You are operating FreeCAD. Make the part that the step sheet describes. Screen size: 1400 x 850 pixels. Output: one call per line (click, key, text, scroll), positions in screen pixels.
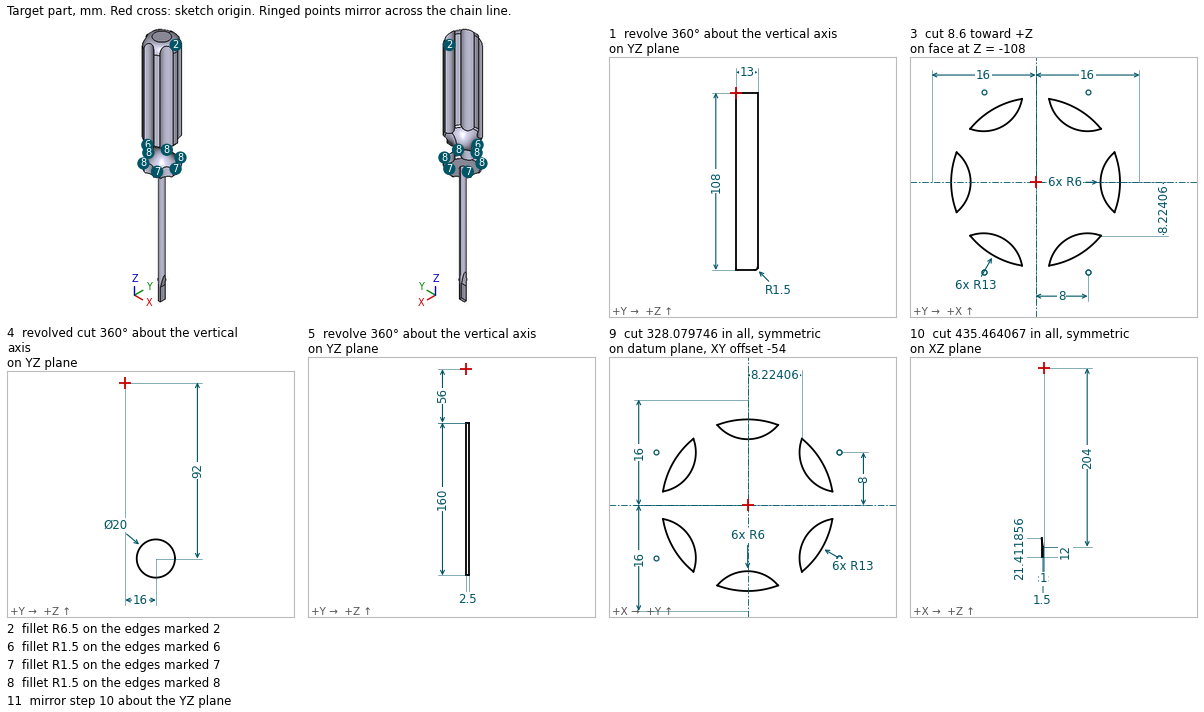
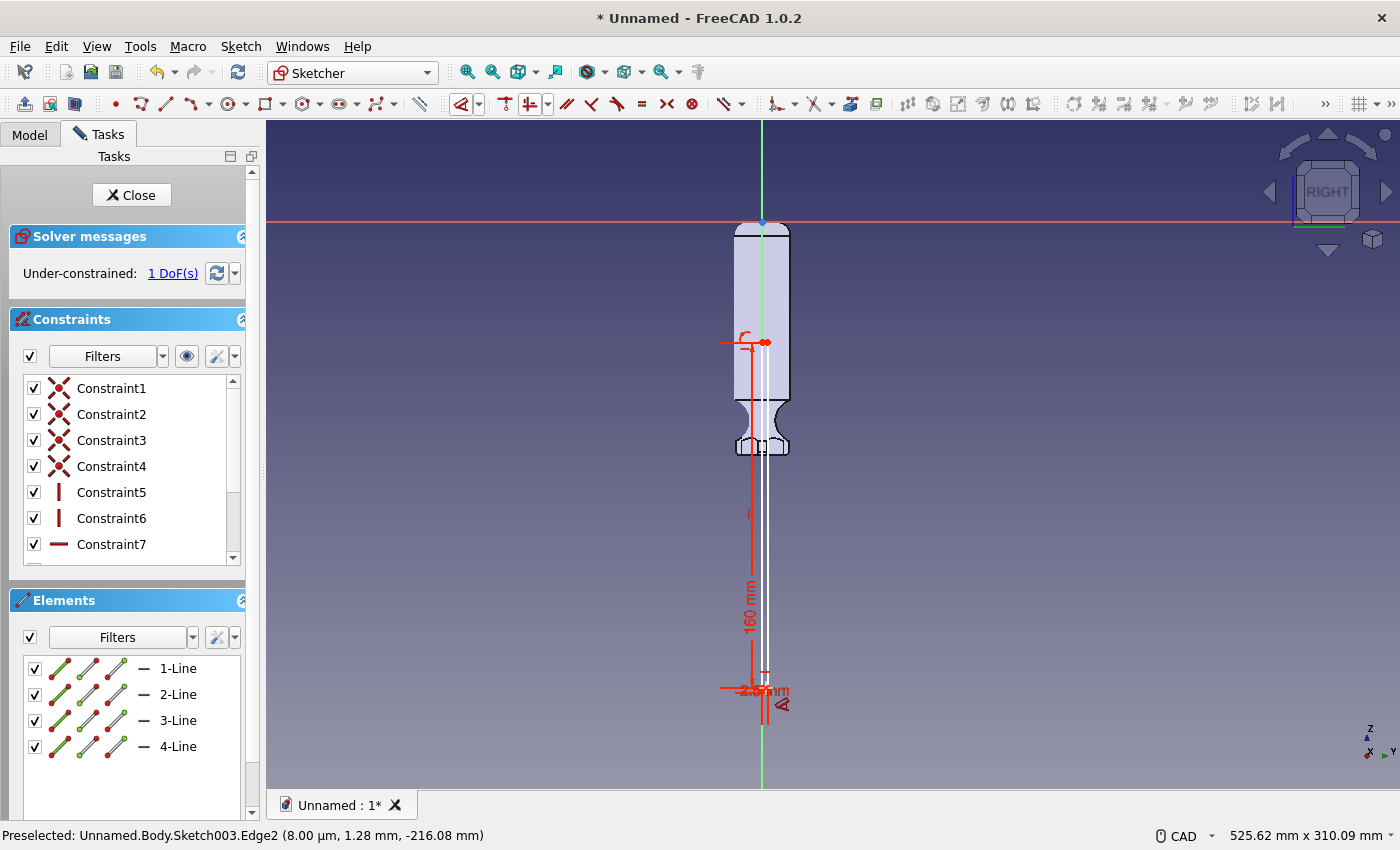
scroll(762, 343, up, 5)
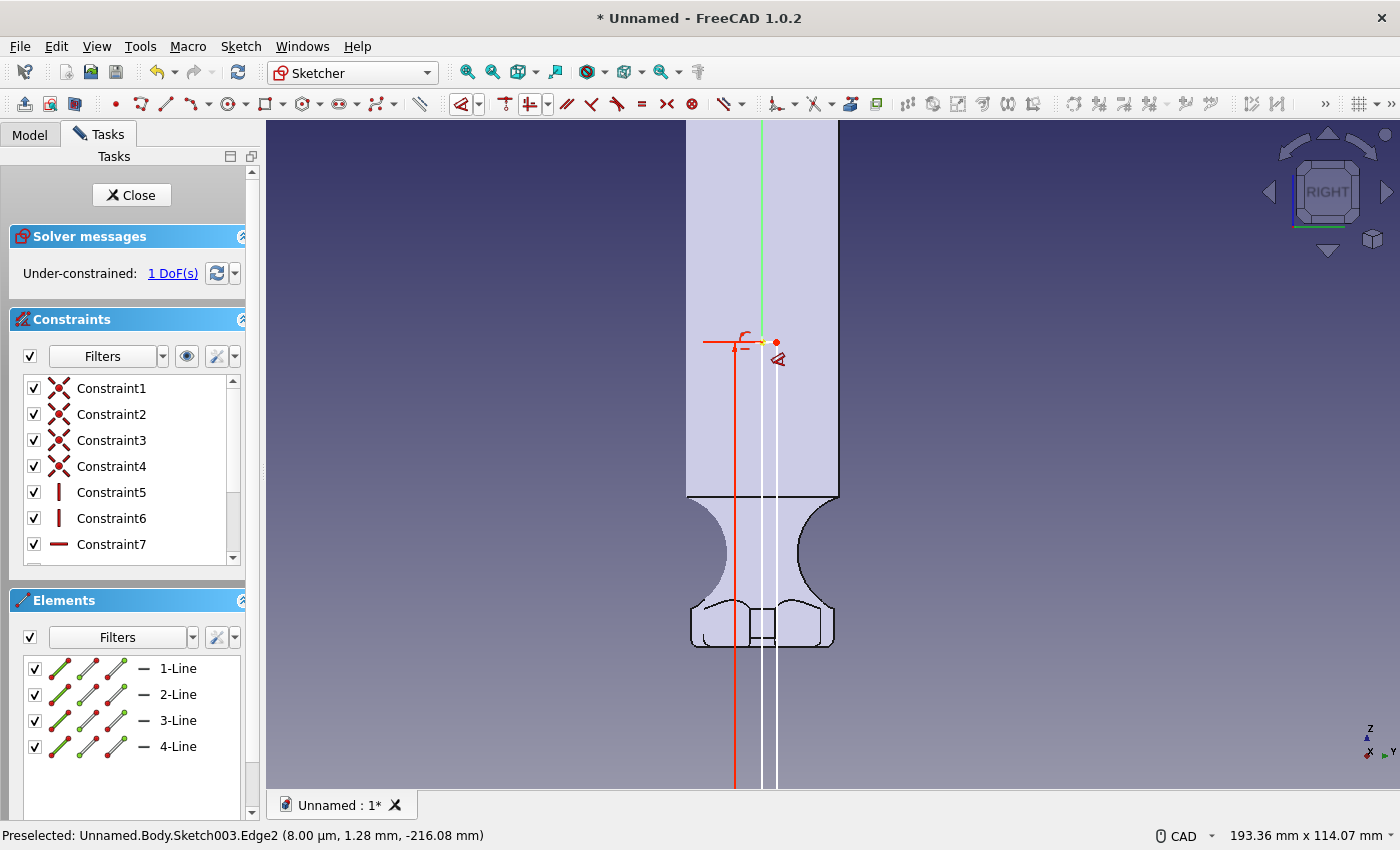
click(762, 342)
click(728, 245)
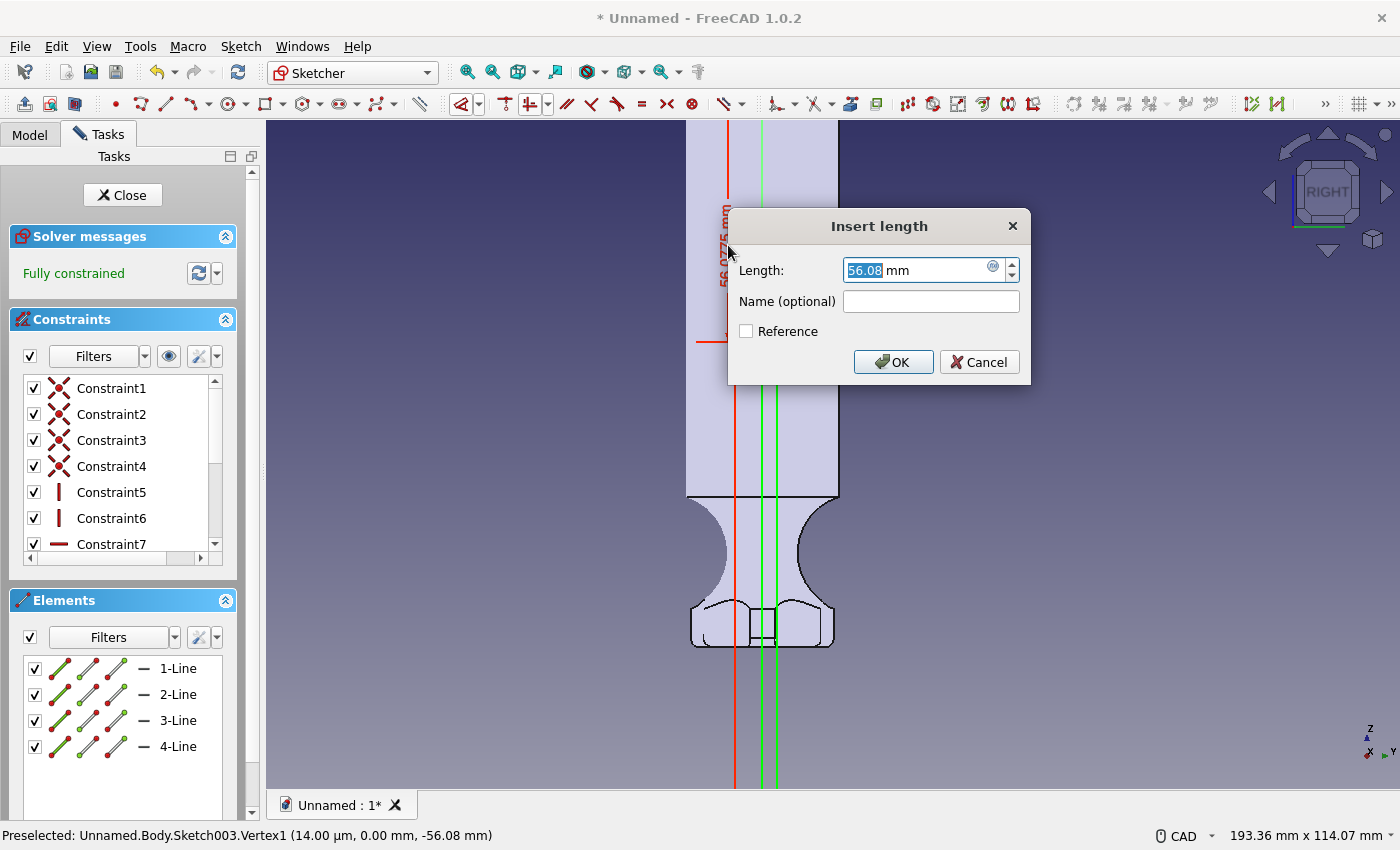
text(56)
key(Return)
key(Escape)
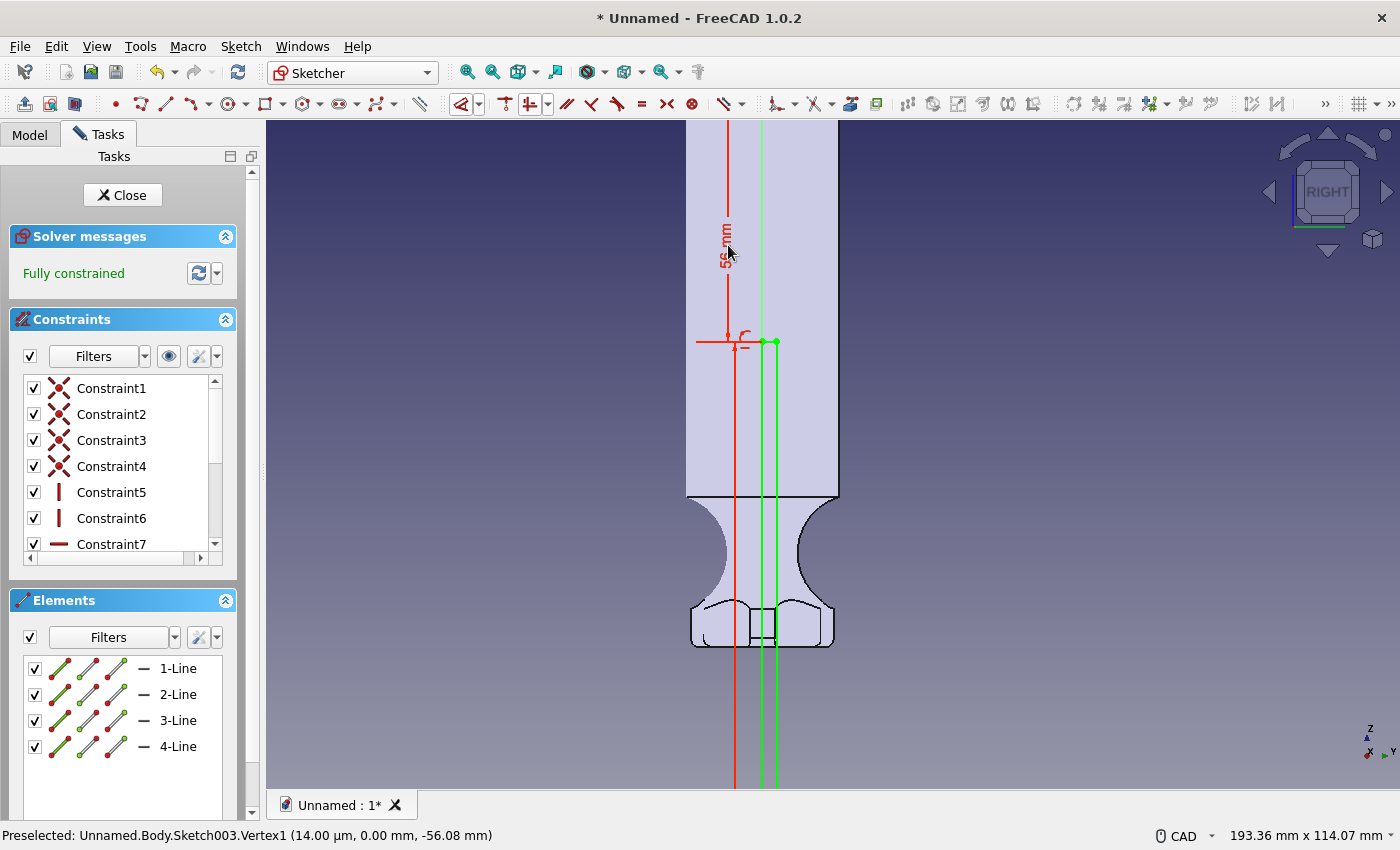
click(123, 195)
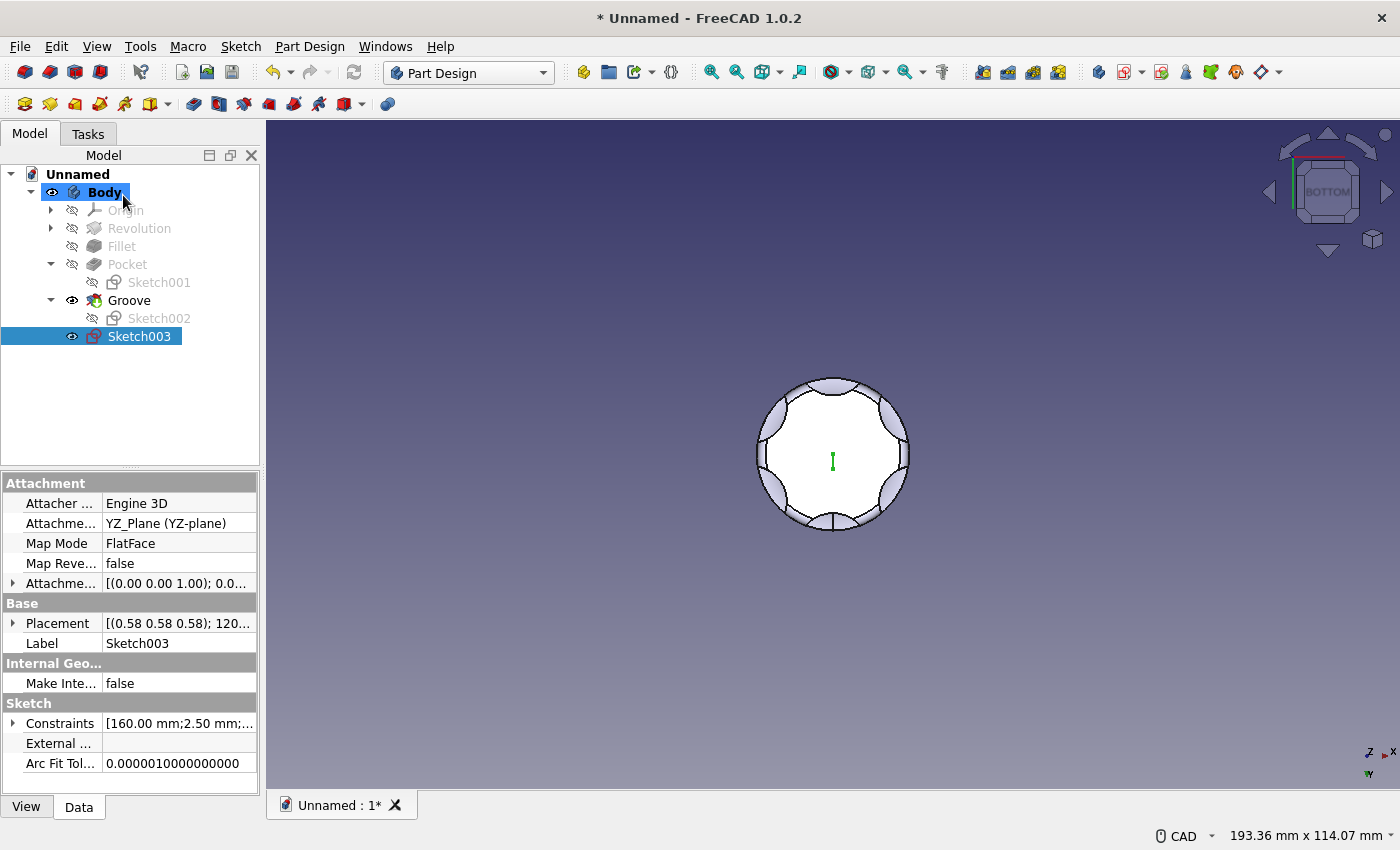
click(50, 104)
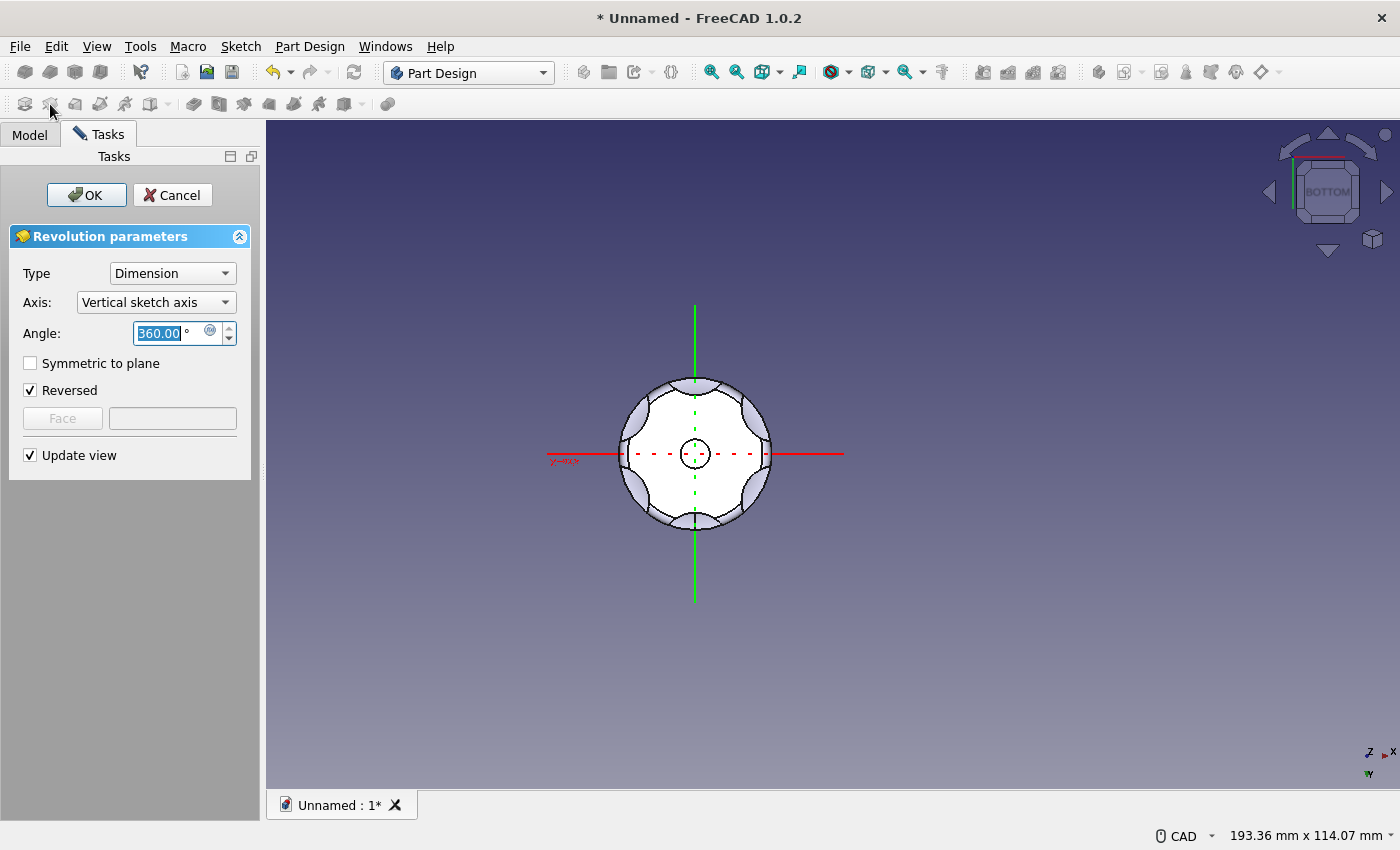
click(87, 195)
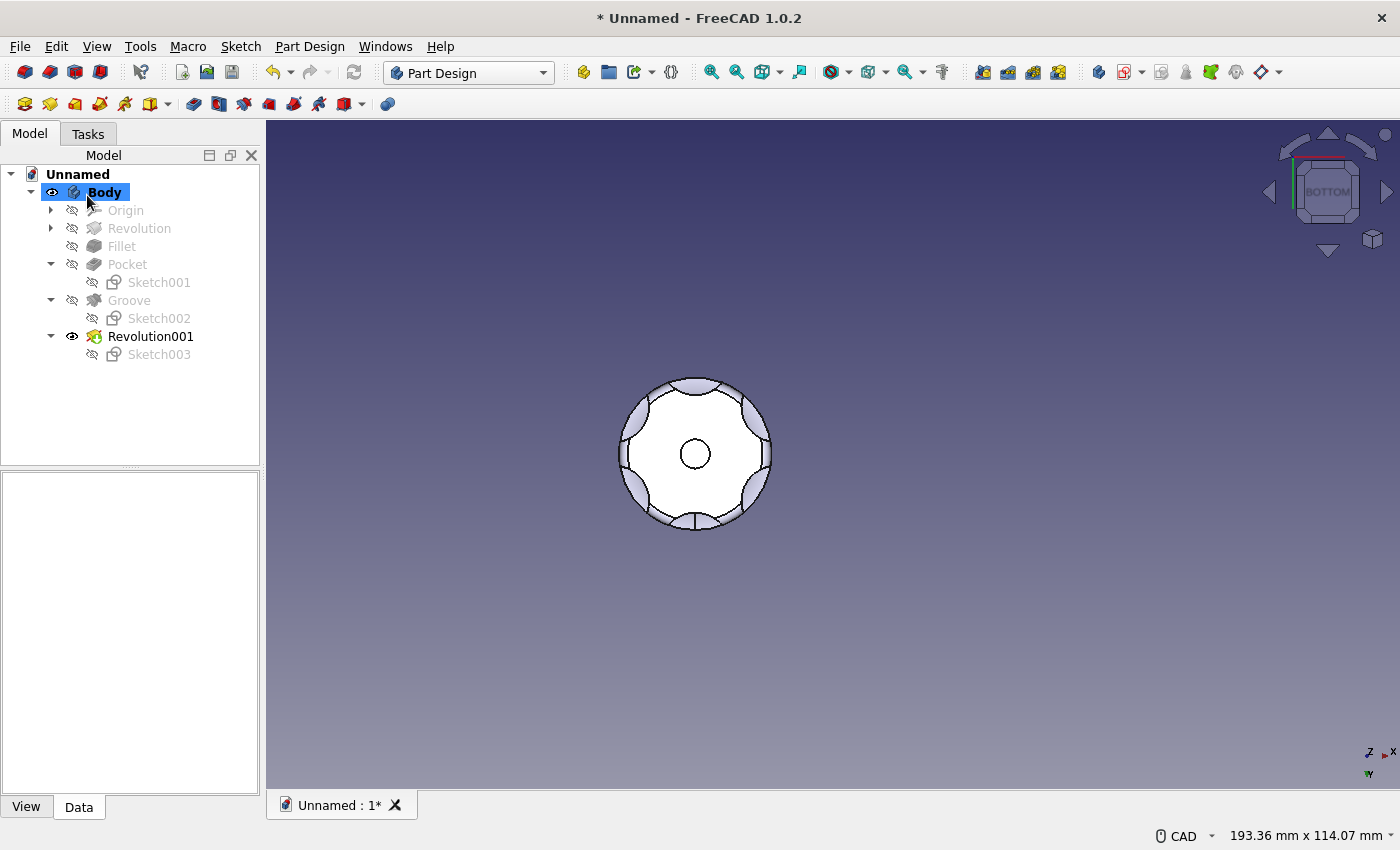
click(712, 72)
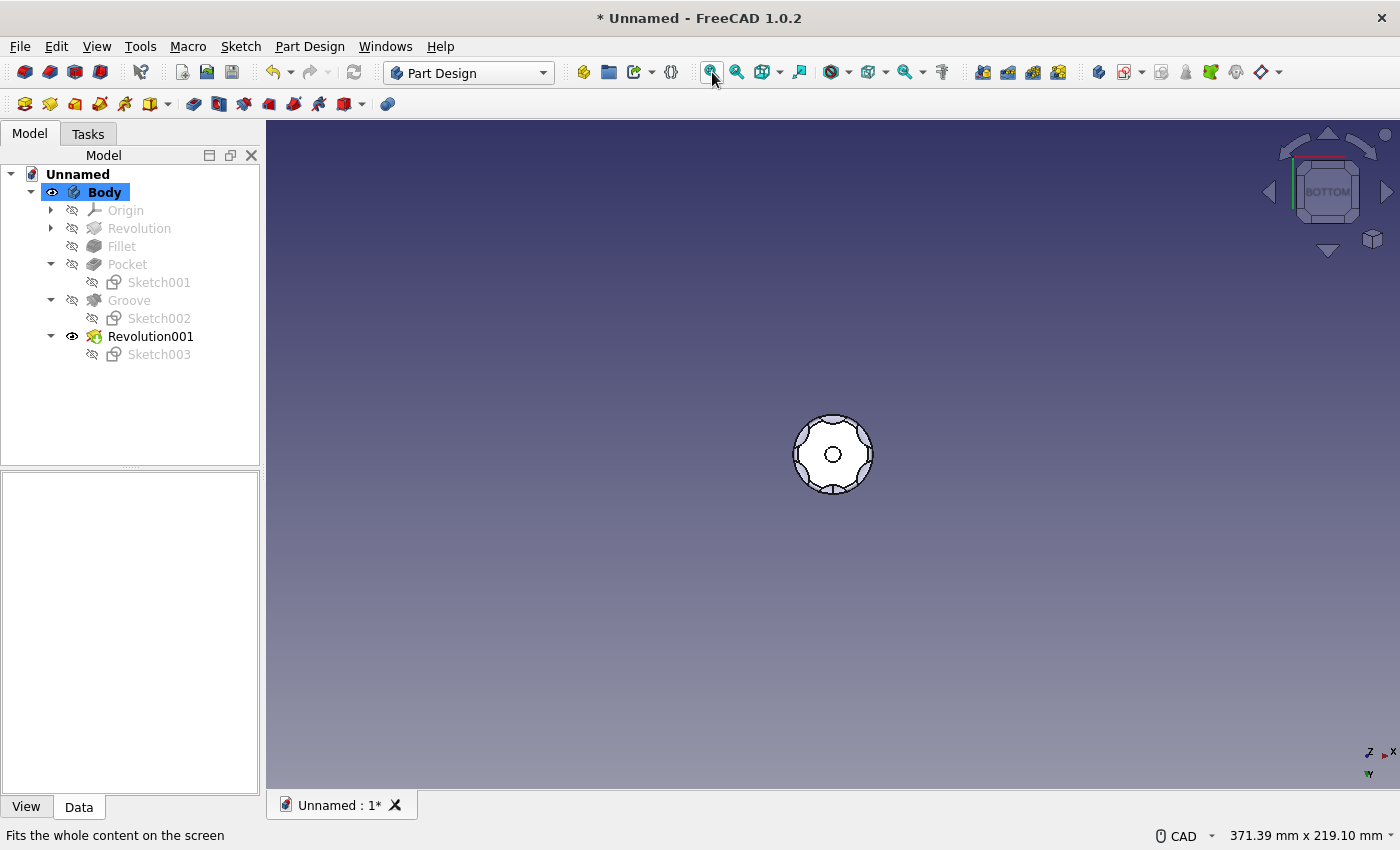
key(0)